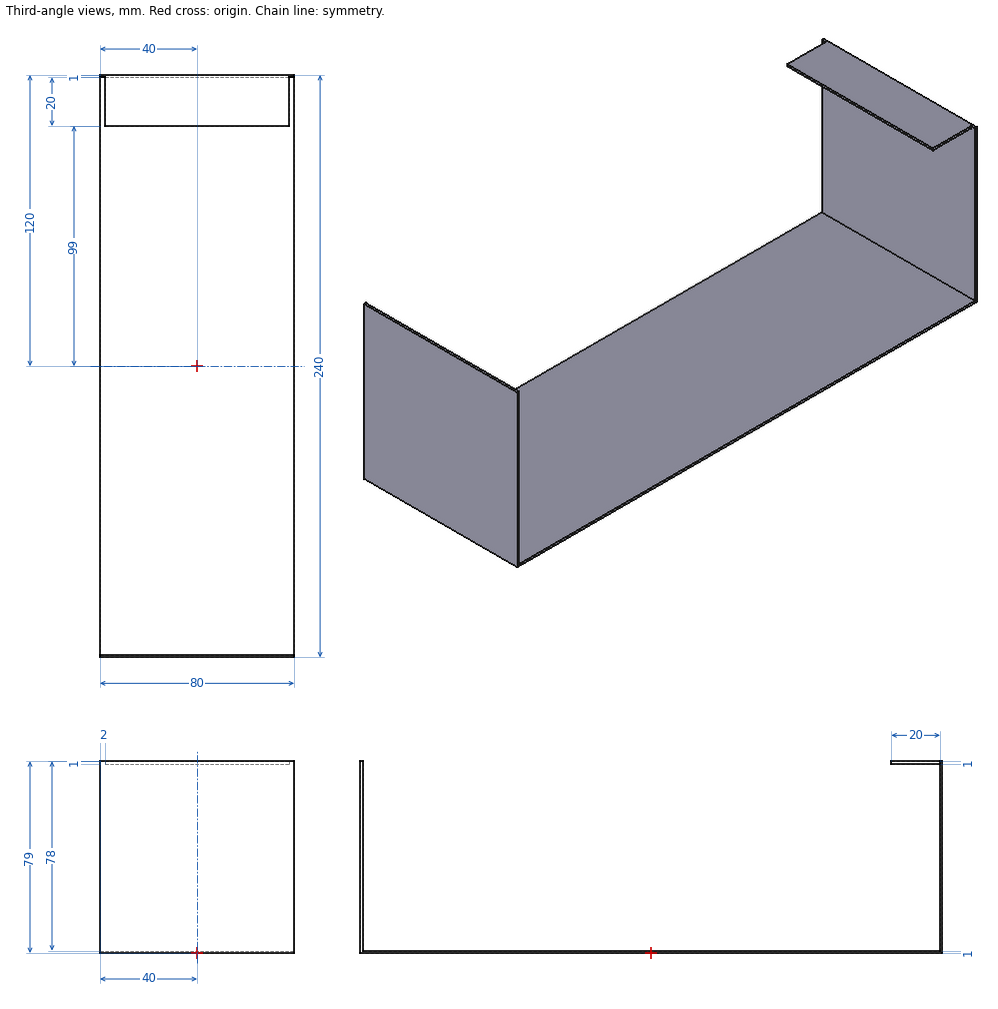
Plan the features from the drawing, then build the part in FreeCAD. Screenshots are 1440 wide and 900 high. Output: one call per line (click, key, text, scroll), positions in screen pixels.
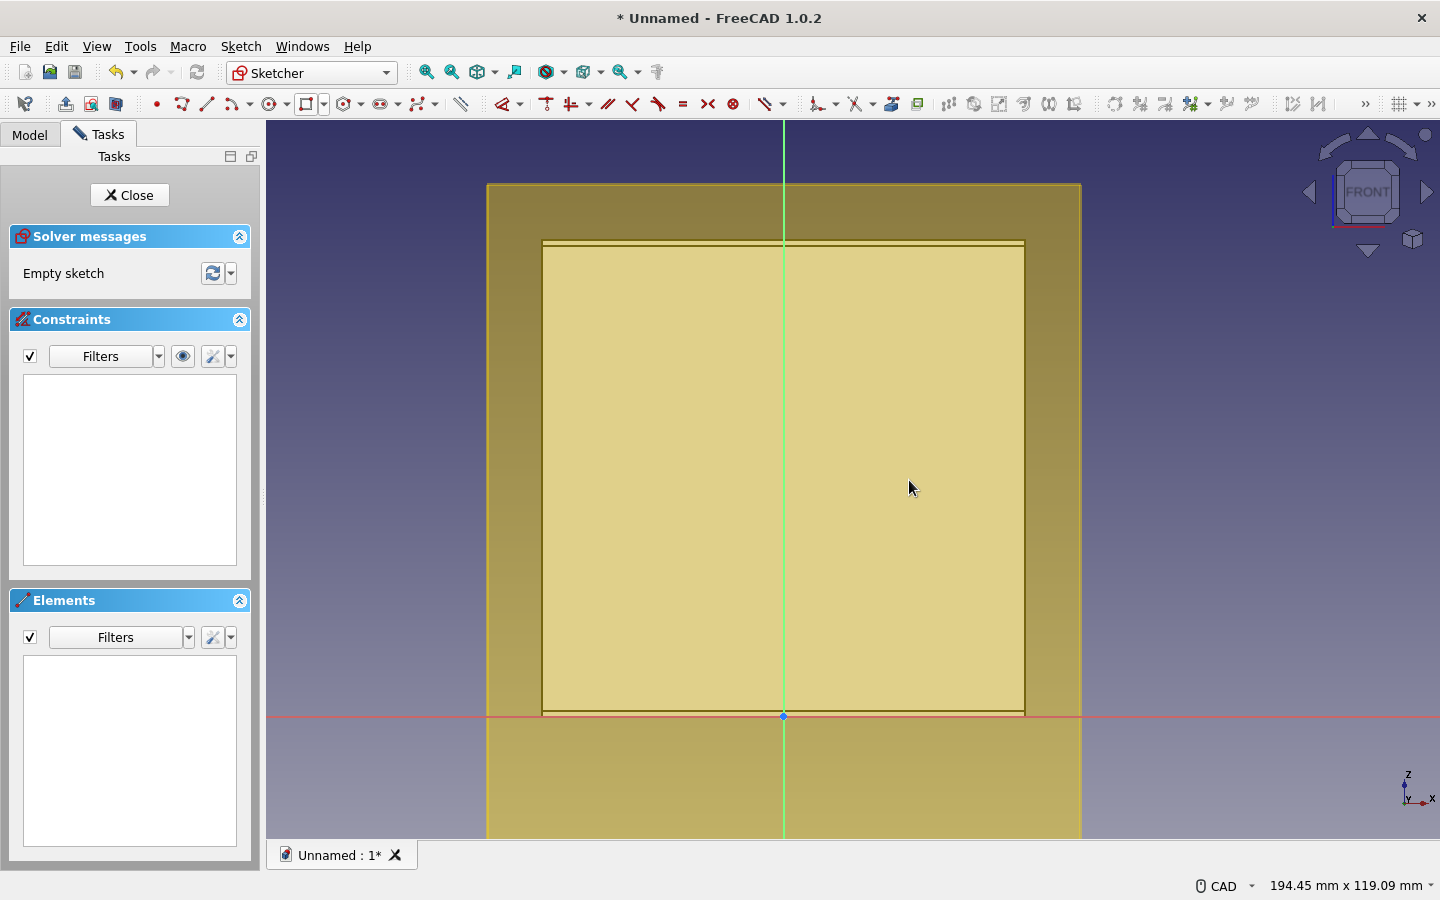
key(g)
key(r)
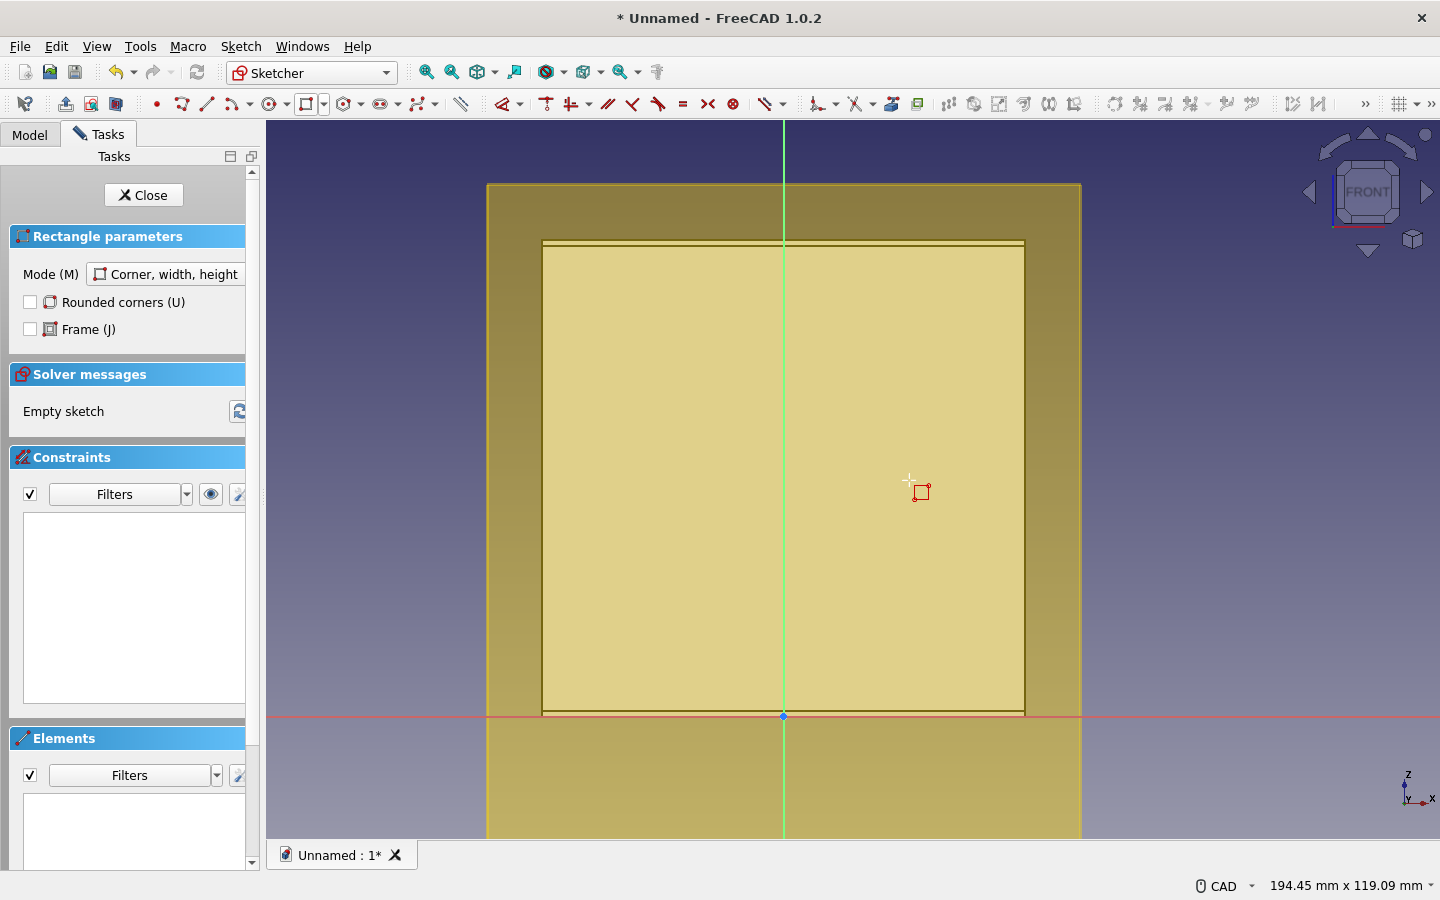
scroll(542, 240, up, 5)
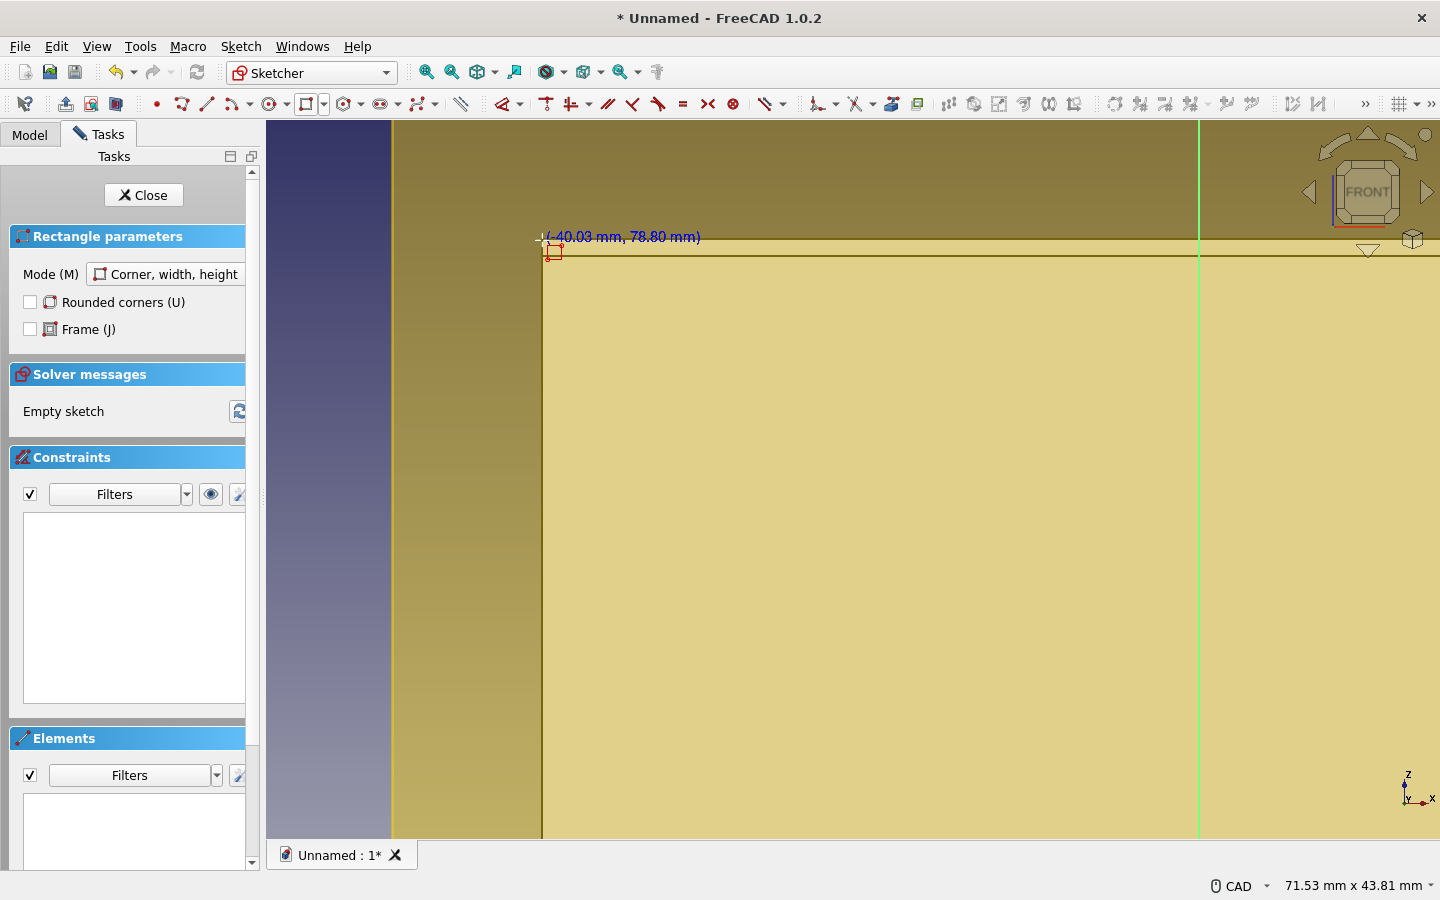
click(542, 239)
click(575, 256)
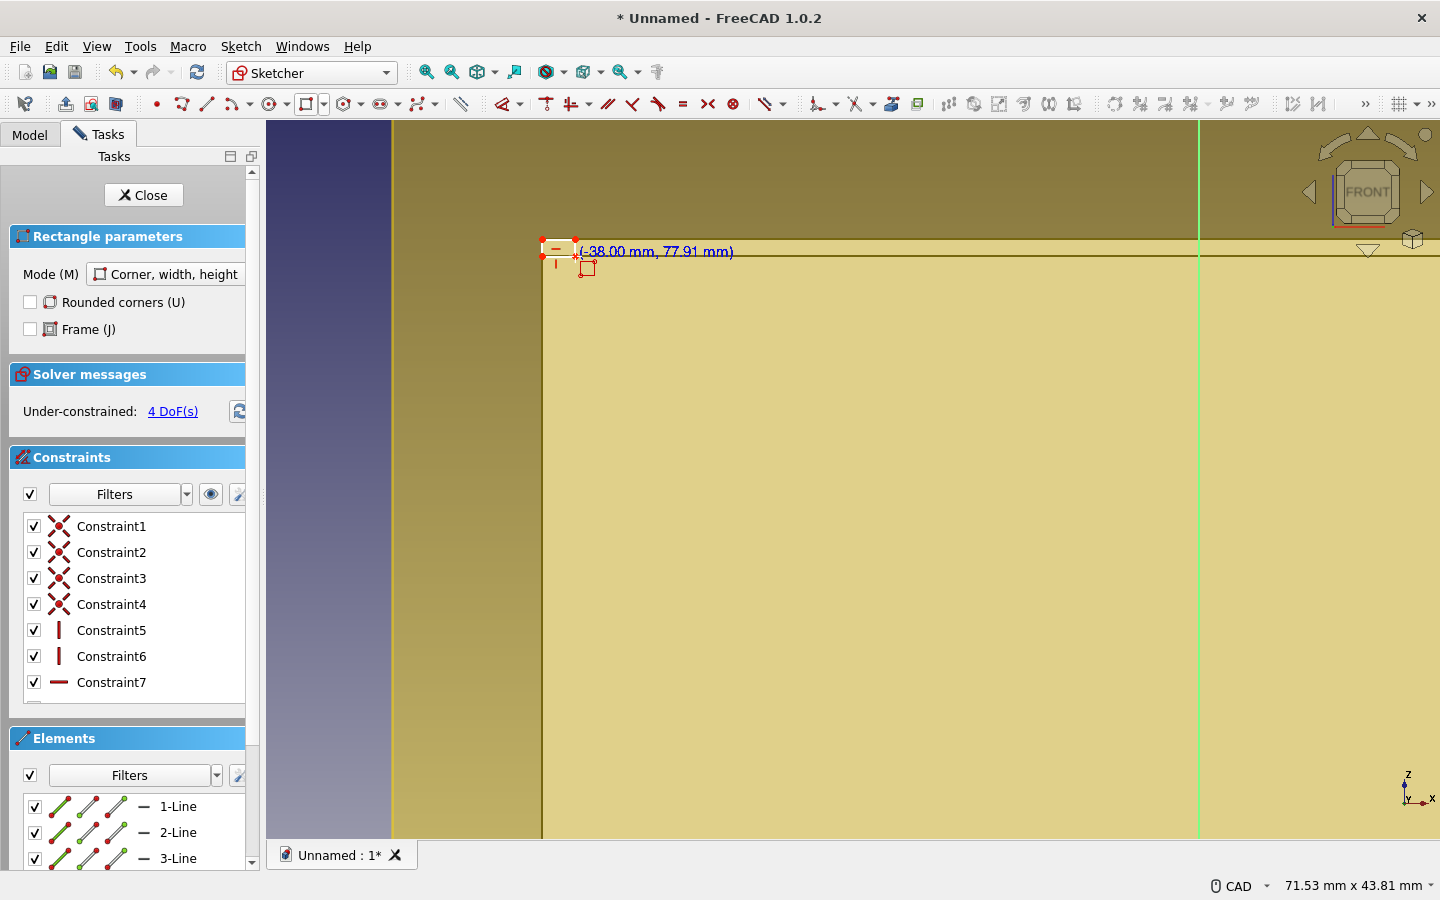
scroll(544, 242, down, 5)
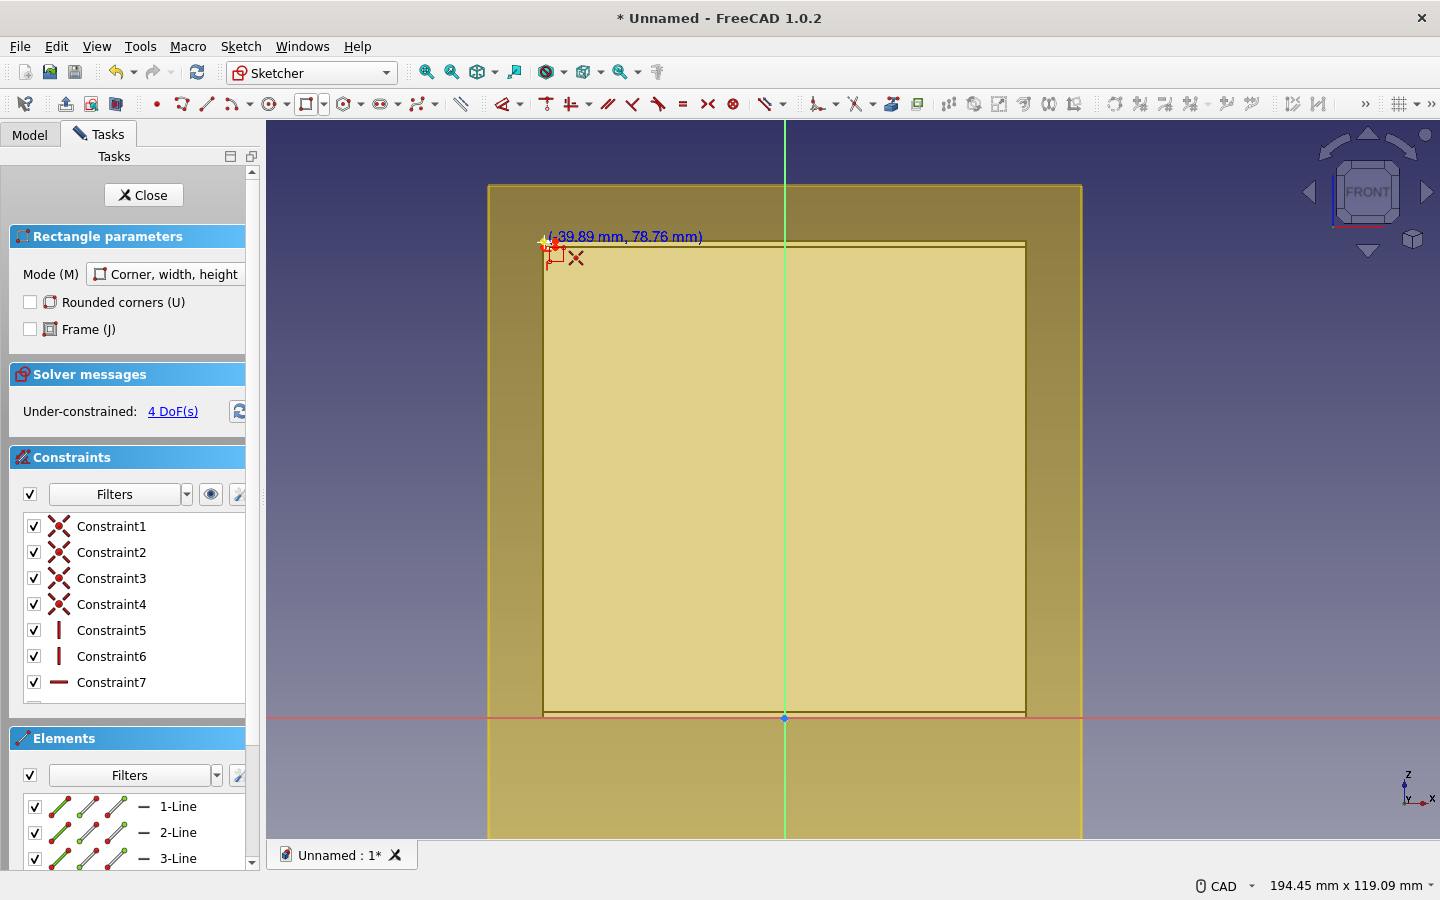
scroll(1014, 241, up, 5)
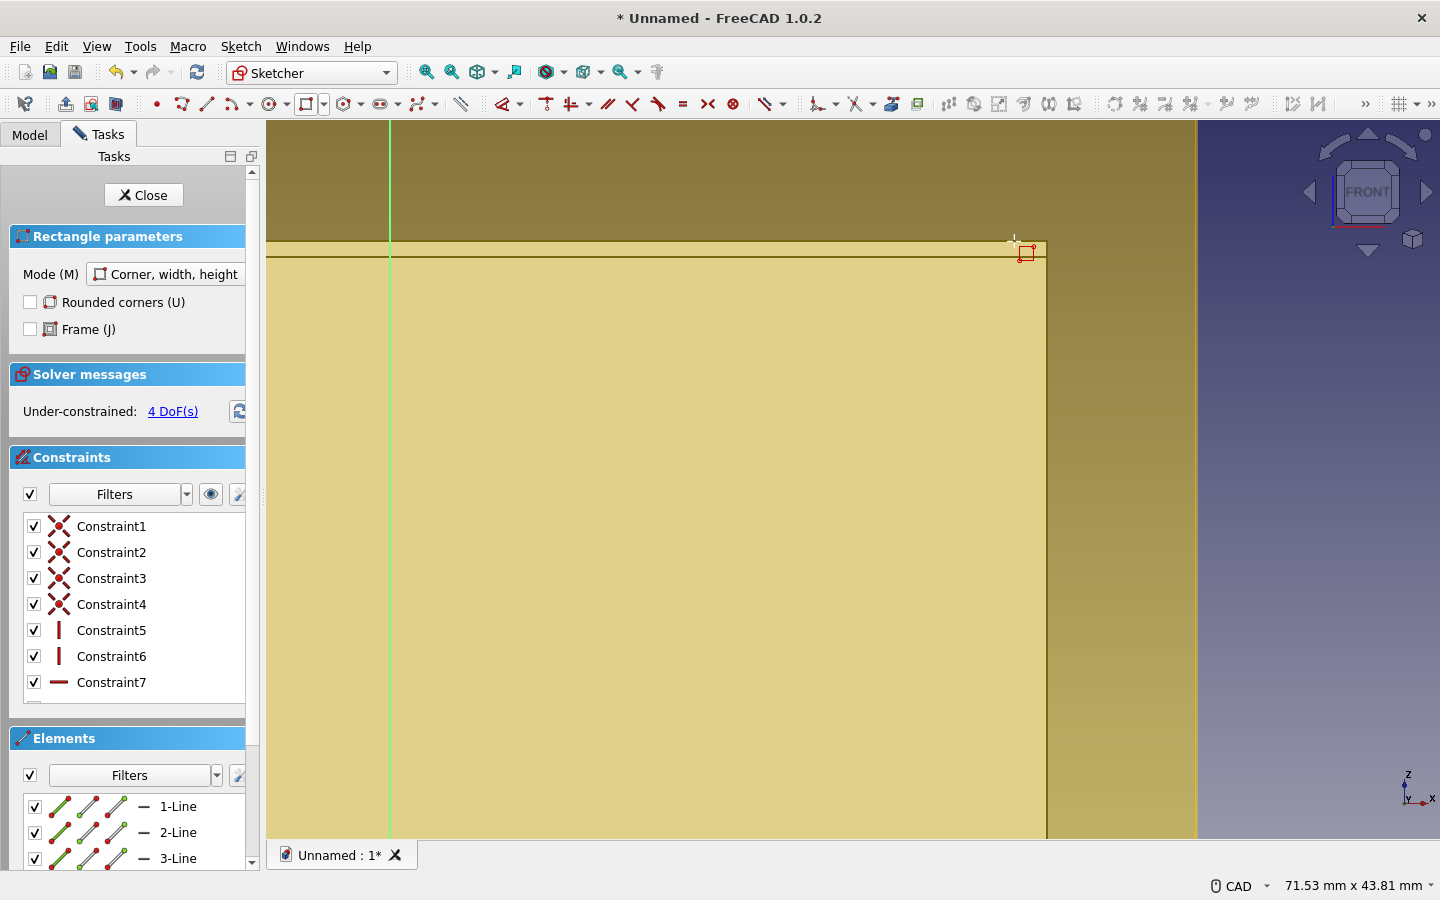
click(1014, 241)
click(1047, 257)
key(Escape)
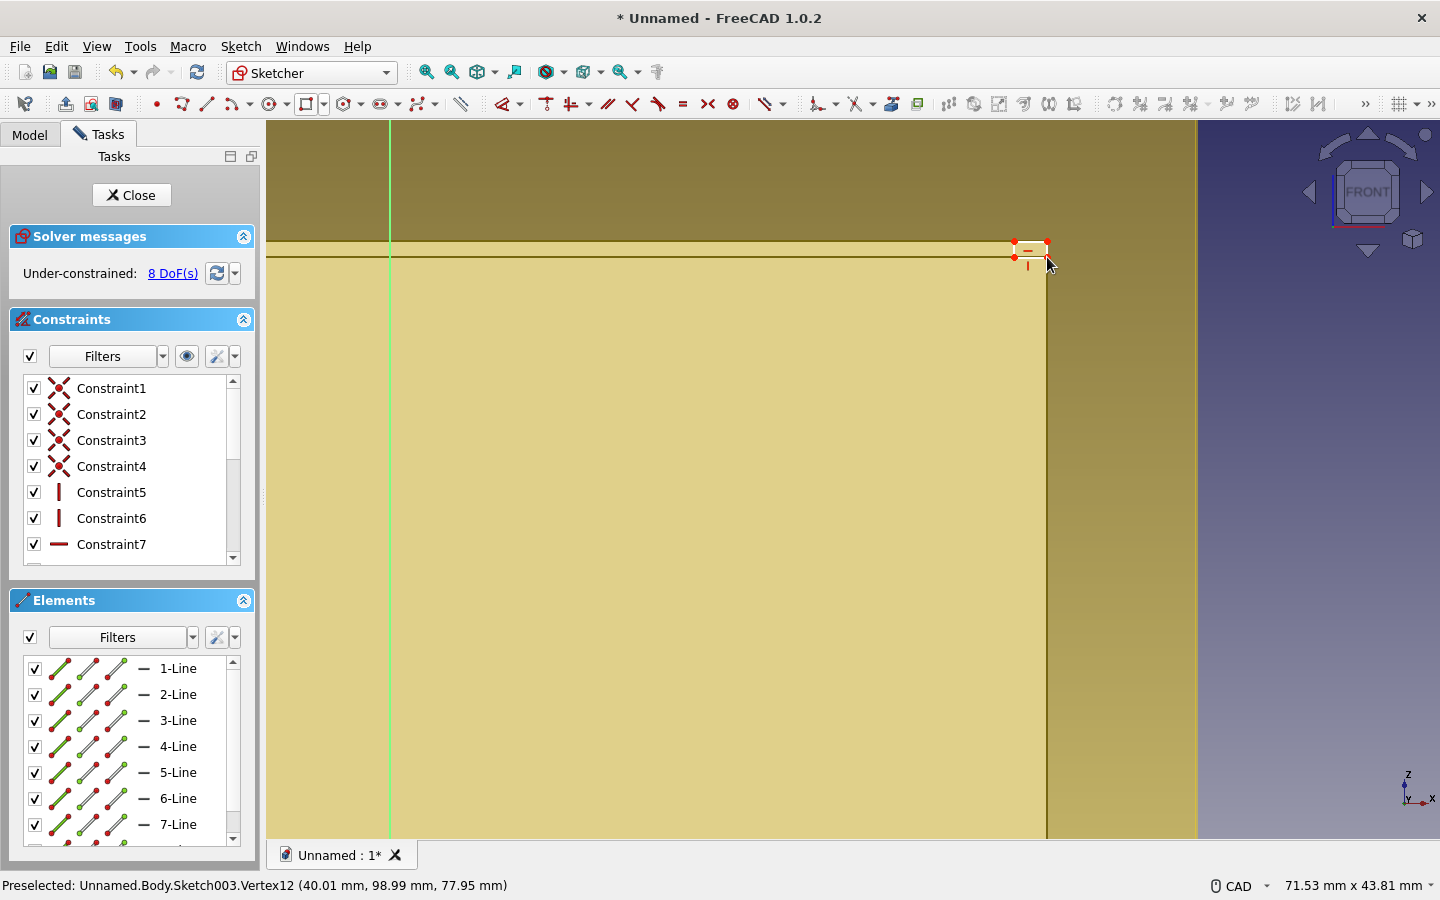
scroll(1014, 241, down, 5)